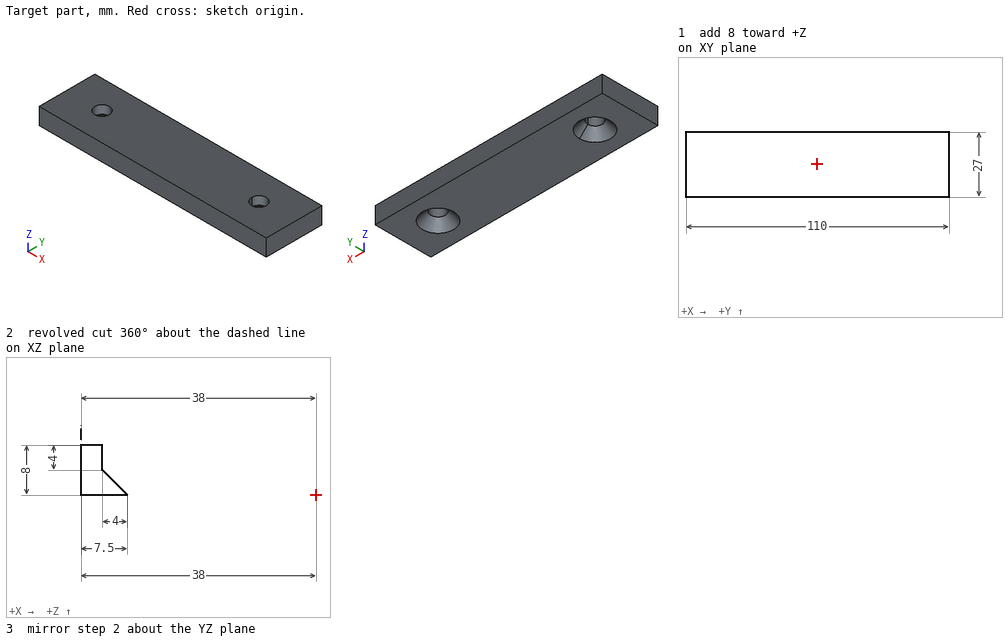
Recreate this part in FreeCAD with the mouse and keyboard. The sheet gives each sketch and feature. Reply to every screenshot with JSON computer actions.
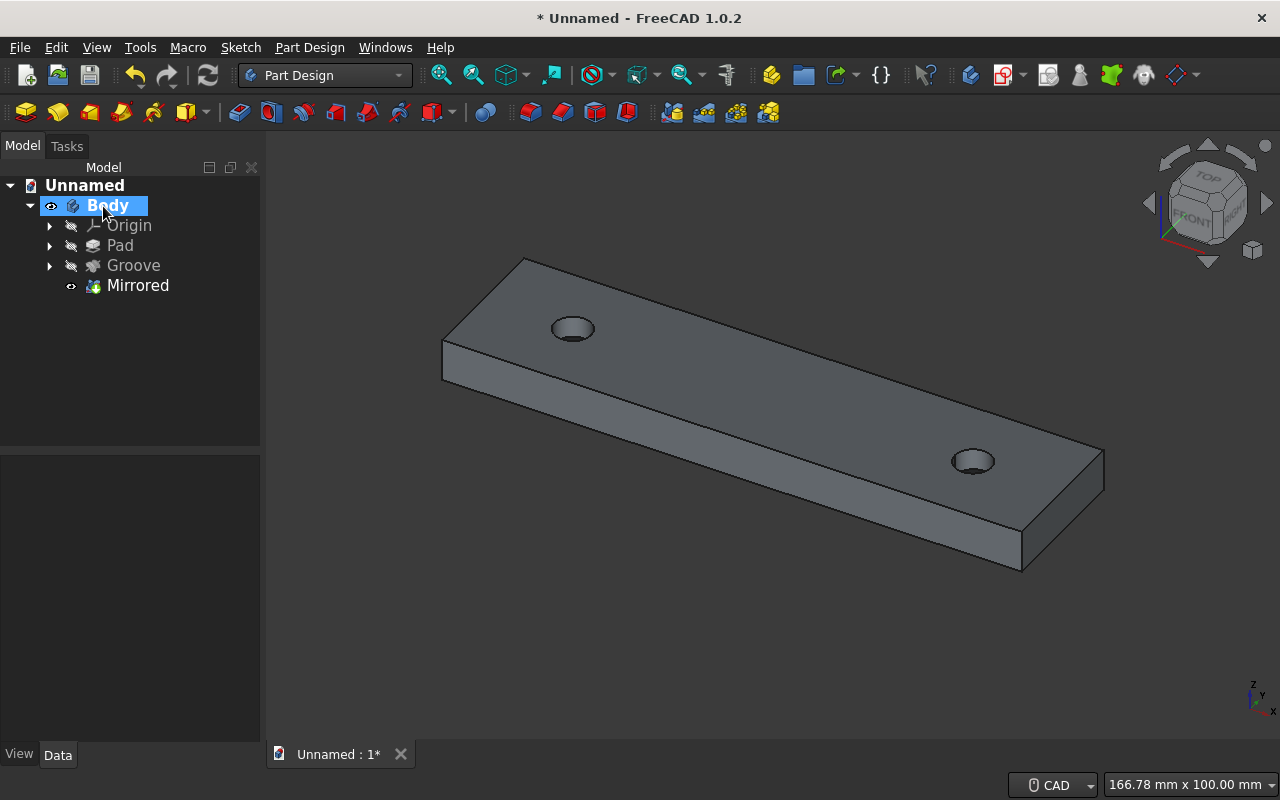
{"action": "key", "text": "0"}